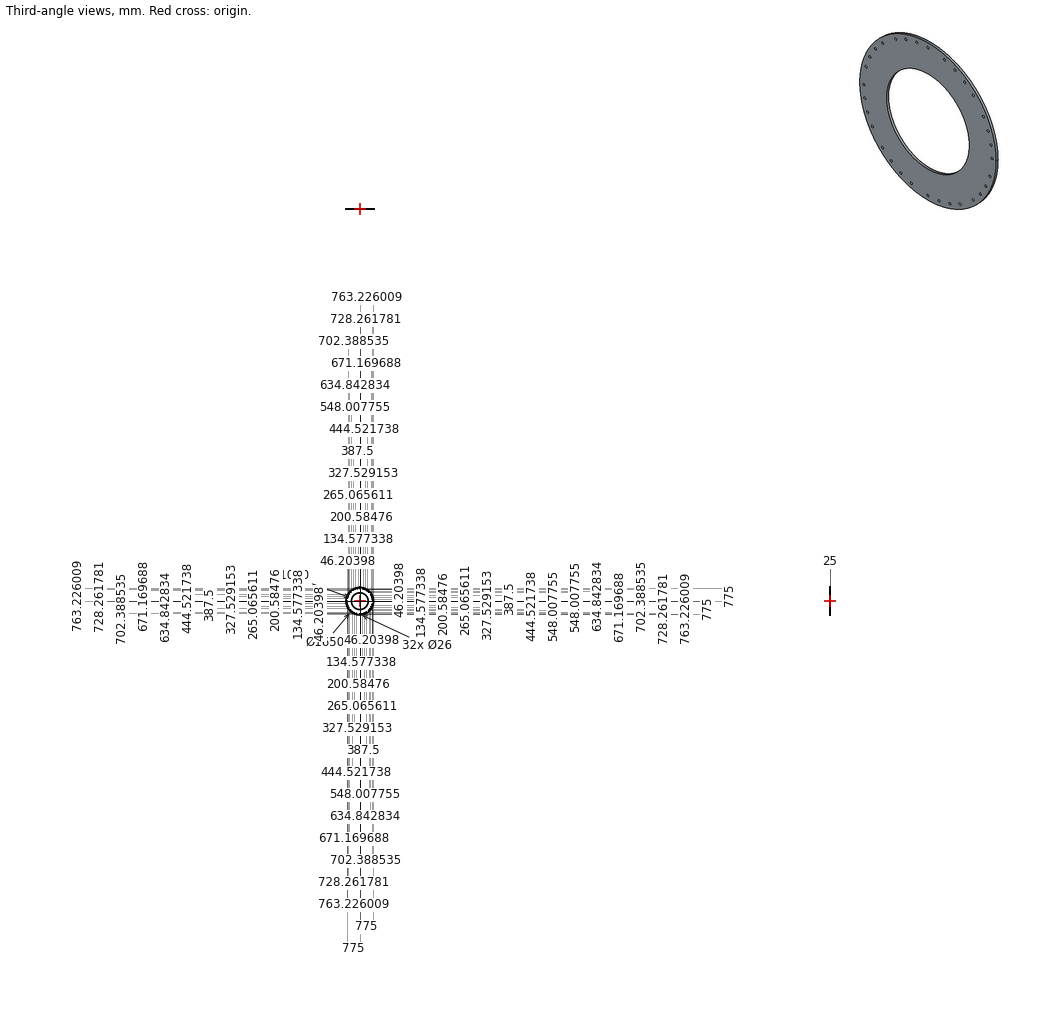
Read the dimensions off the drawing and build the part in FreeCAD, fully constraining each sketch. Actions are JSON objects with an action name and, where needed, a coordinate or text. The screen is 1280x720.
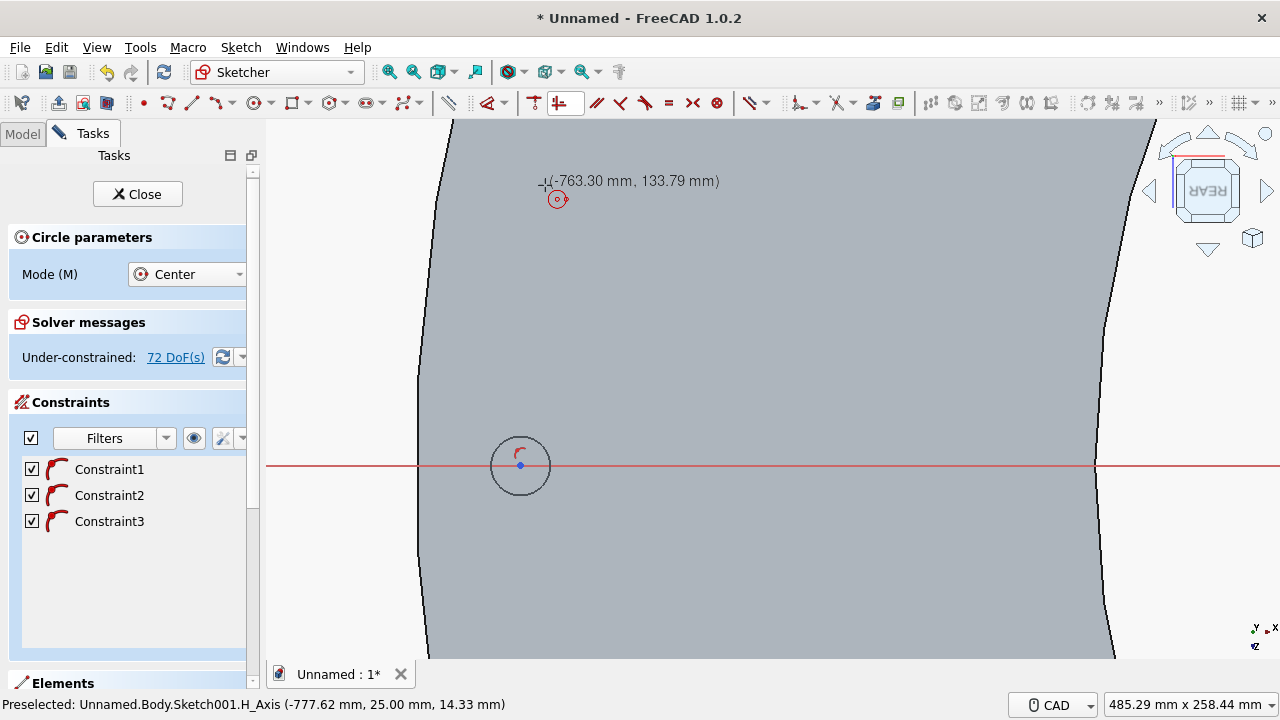
{"action": "scroll", "coordinate": [526, 379], "scroll_direction": "down", "scroll_amount": 11}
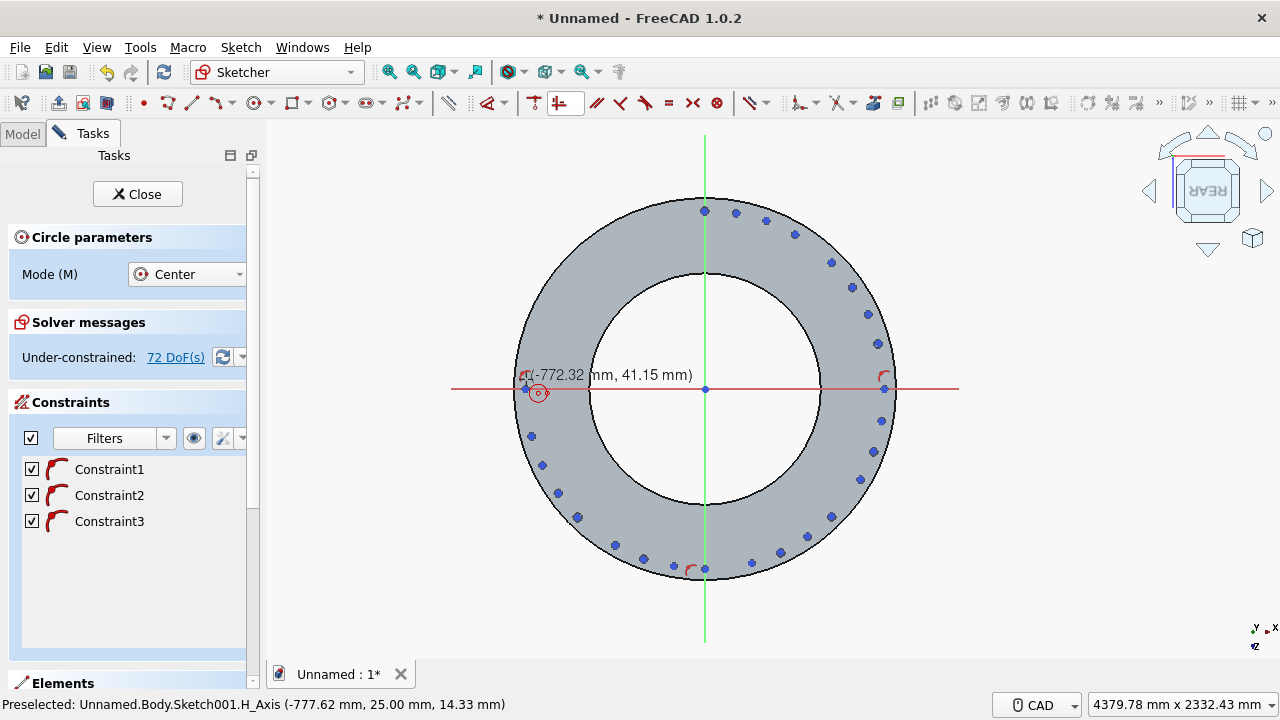
{"action": "left_click", "coordinate": [528, 358]}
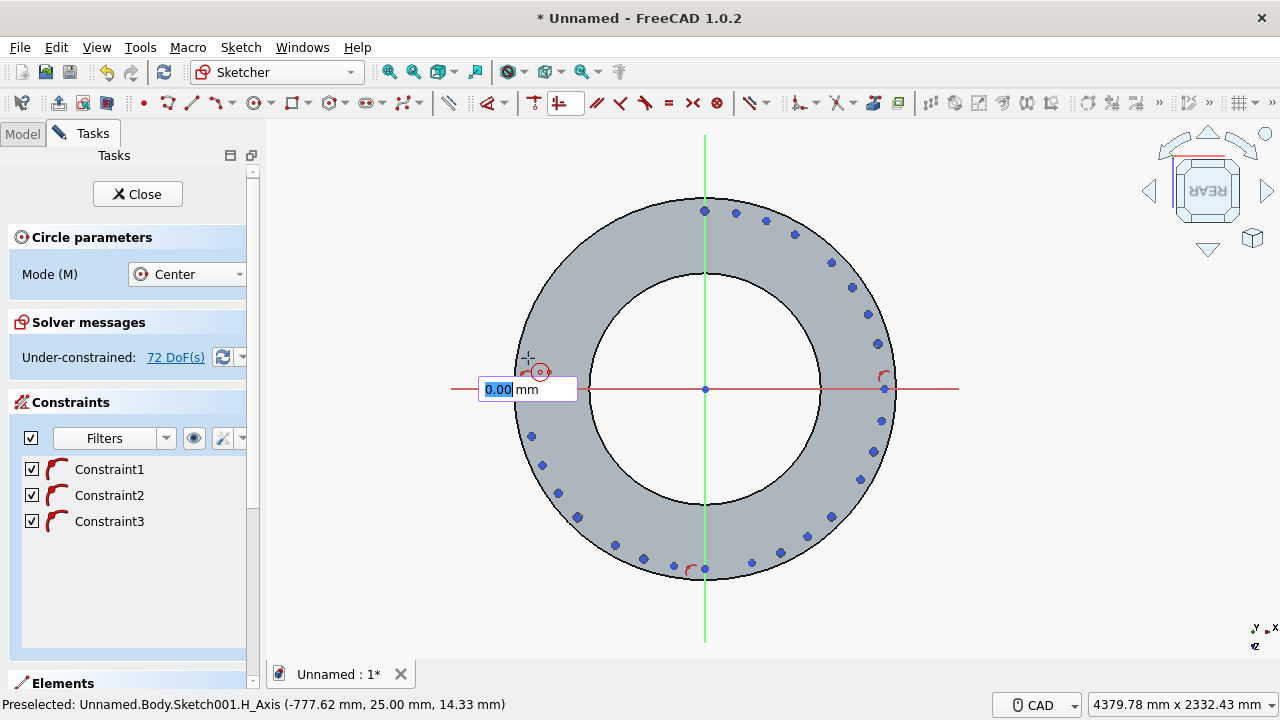
{"action": "scroll", "coordinate": [530, 356], "scroll_direction": "up", "scroll_amount": 9}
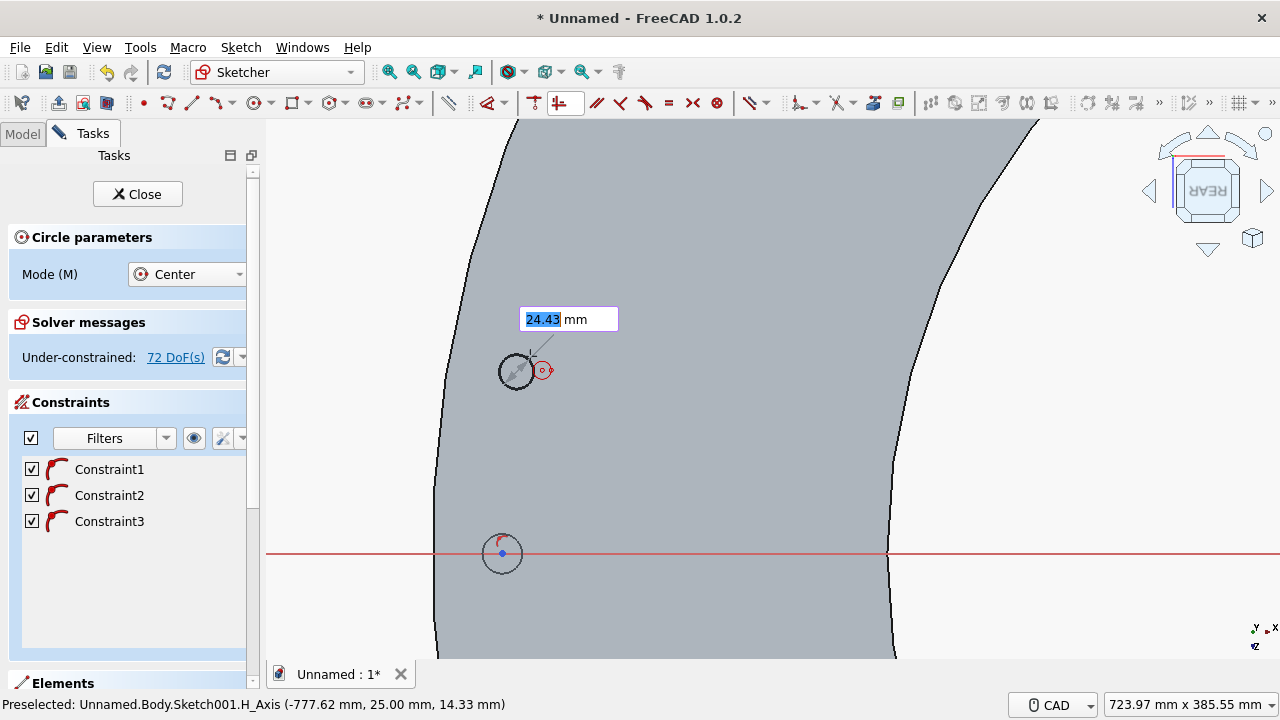
{"action": "left_click", "coordinate": [531, 352]}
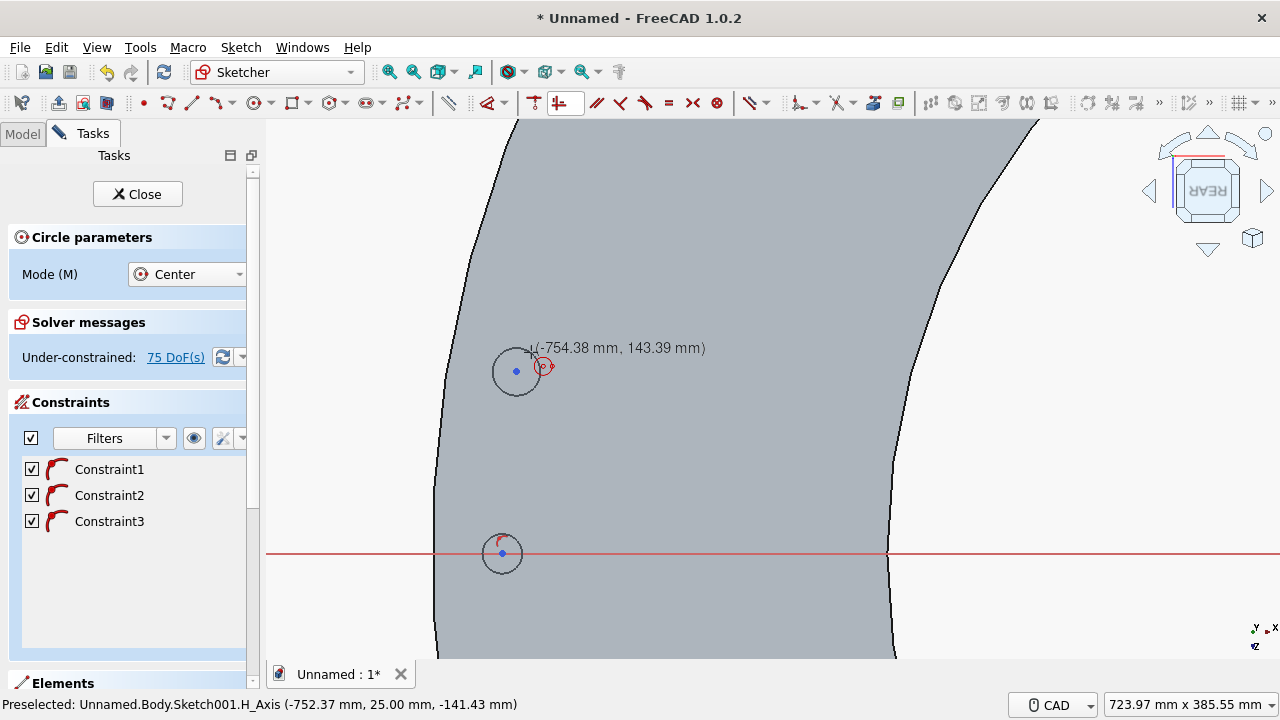
{"action": "scroll", "coordinate": [568, 183], "scroll_direction": "up", "scroll_amount": 2}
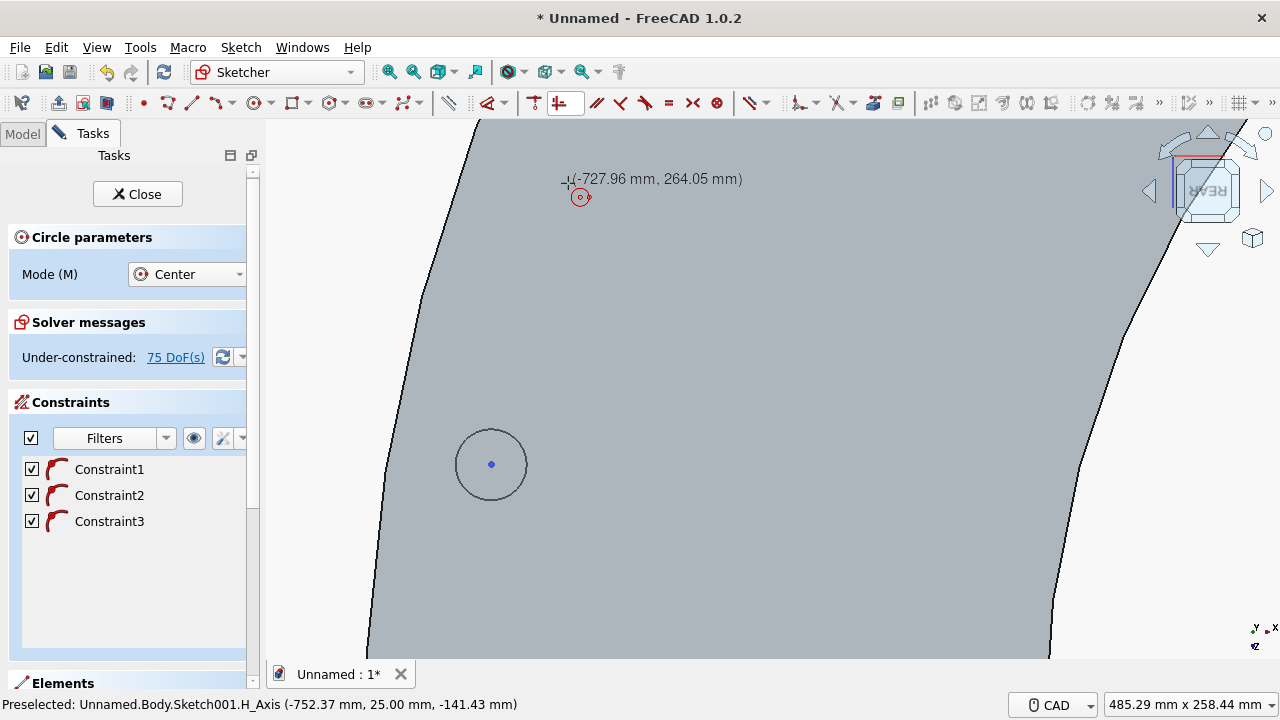
{"action": "scroll", "coordinate": [532, 346], "scroll_direction": "down", "scroll_amount": 11}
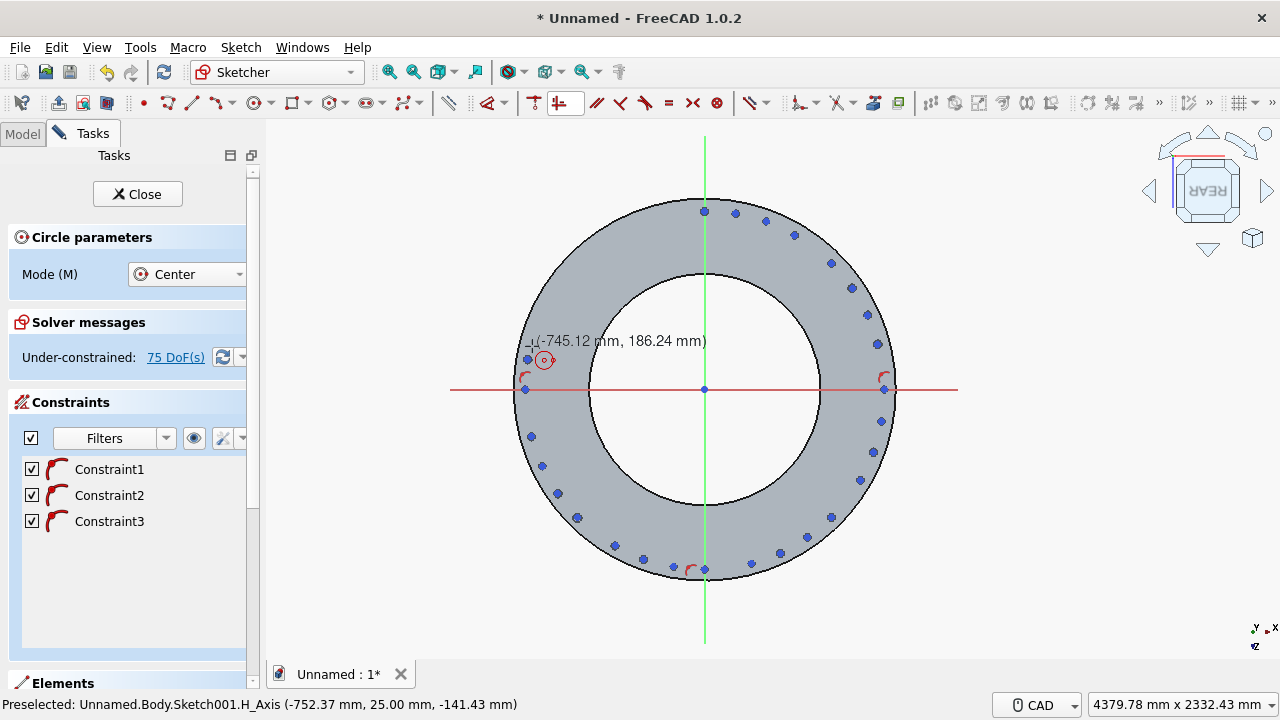
{"action": "left_click", "coordinate": [536, 328]}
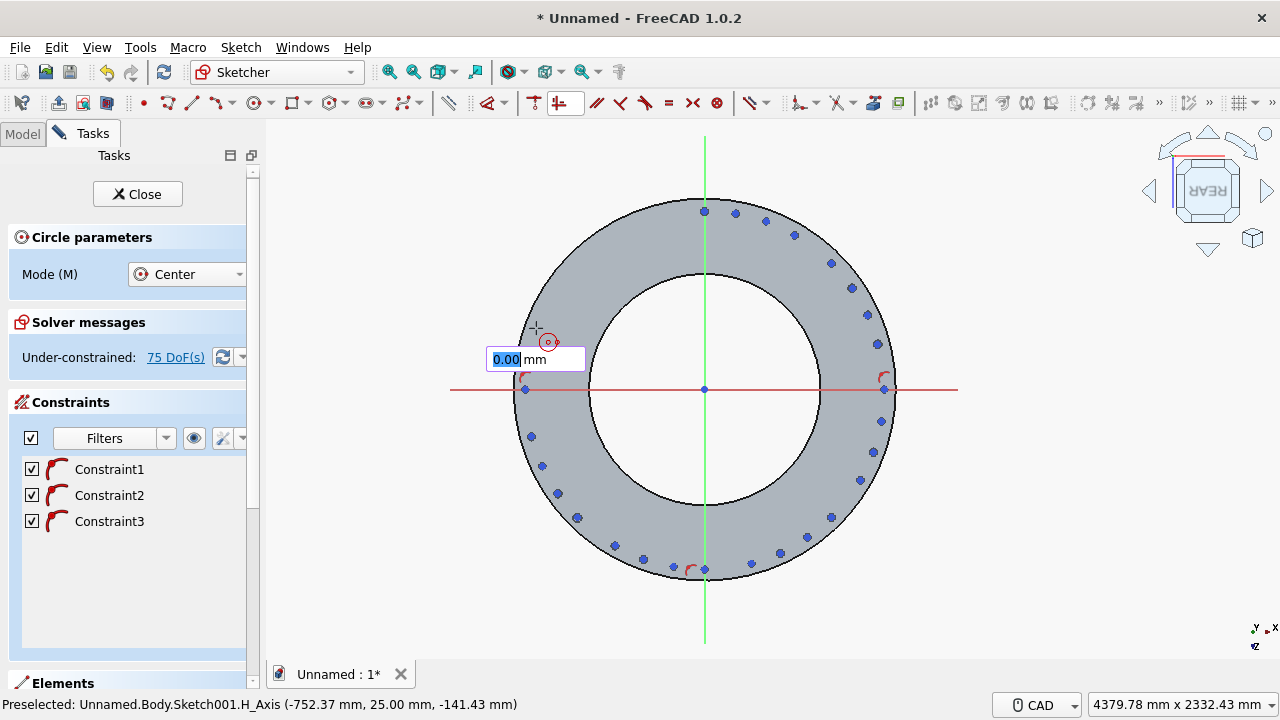
{"action": "scroll", "coordinate": [538, 326], "scroll_direction": "up", "scroll_amount": 9}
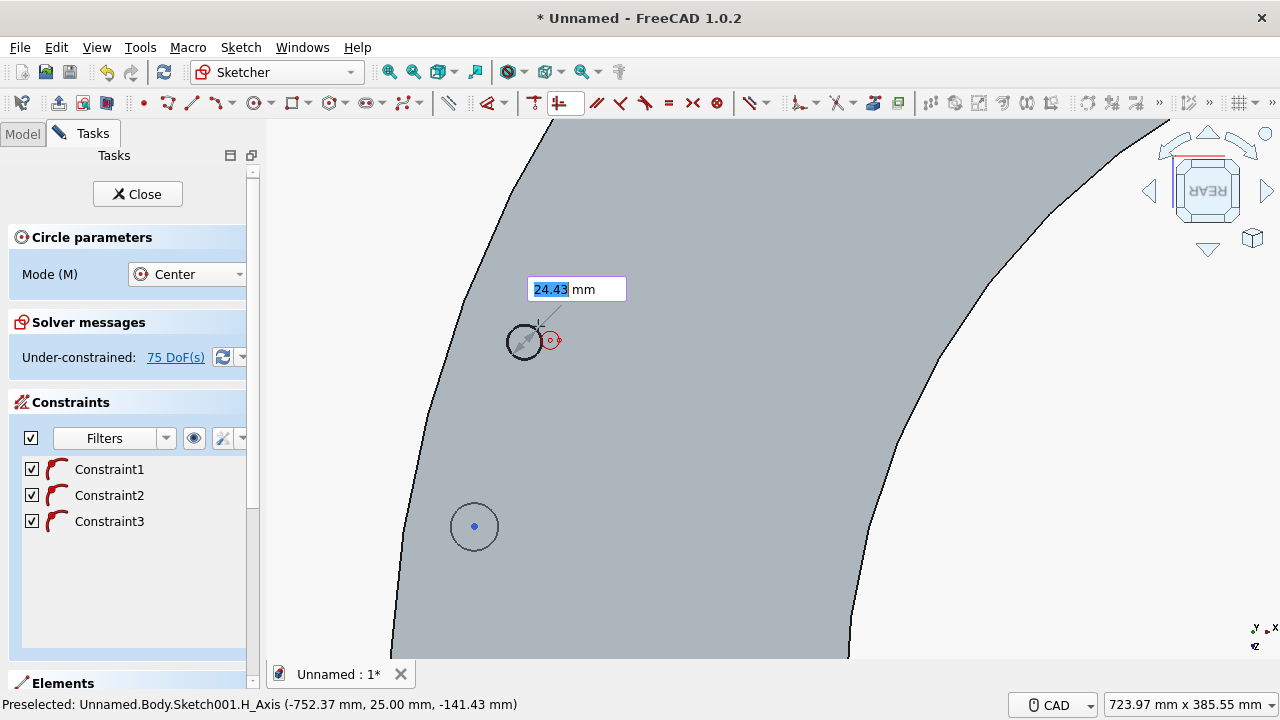
{"action": "left_click", "coordinate": [538, 325]}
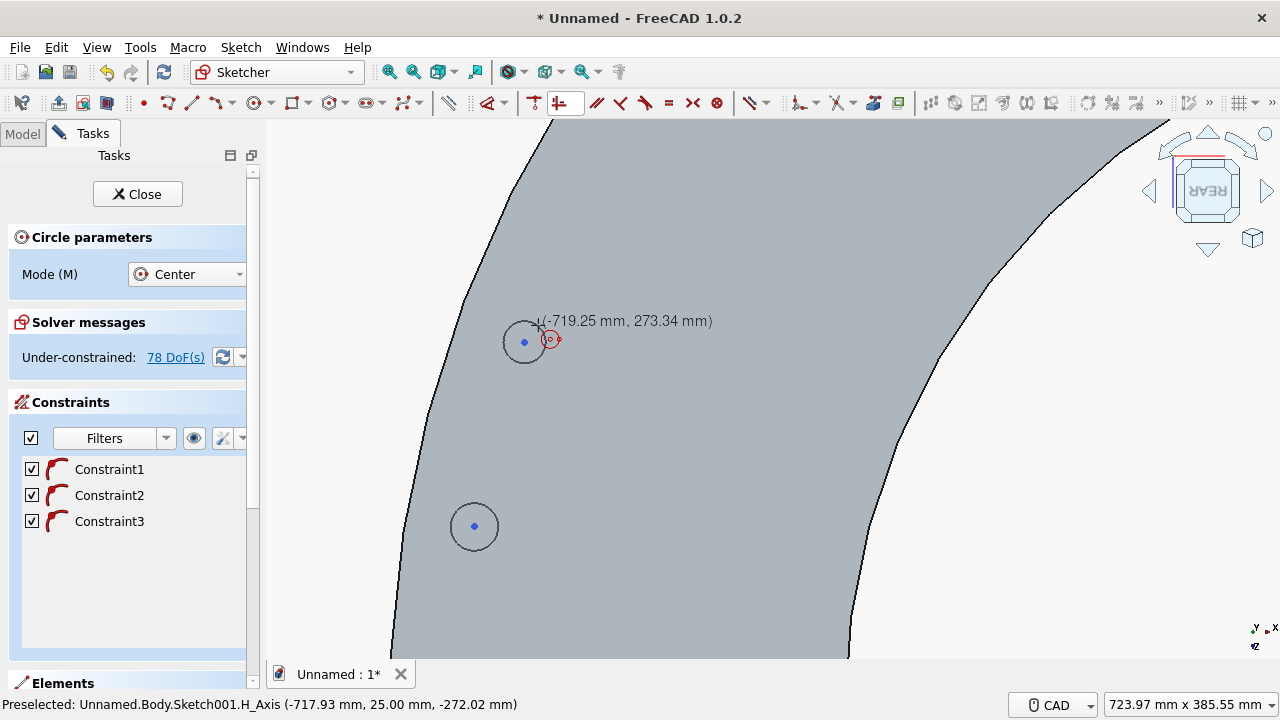
{"action": "scroll", "coordinate": [605, 166], "scroll_direction": "up", "scroll_amount": 2}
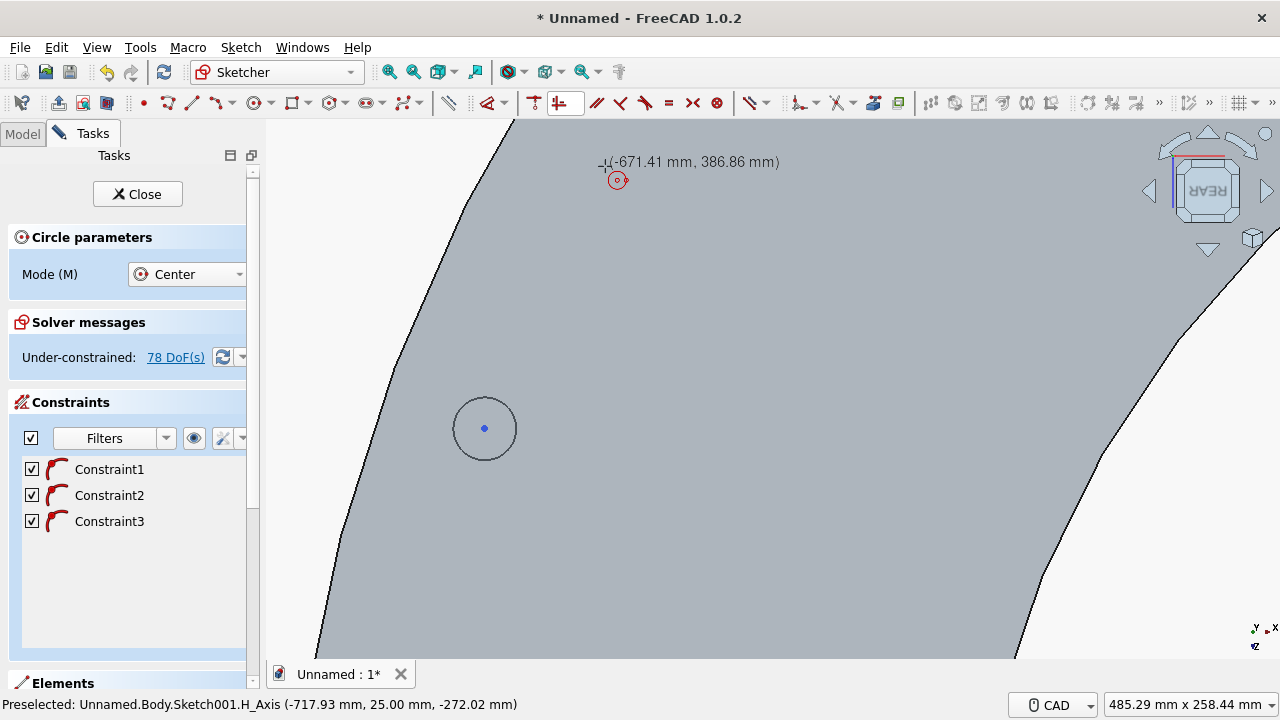
{"action": "scroll", "coordinate": [542, 316], "scroll_direction": "down", "scroll_amount": 11}